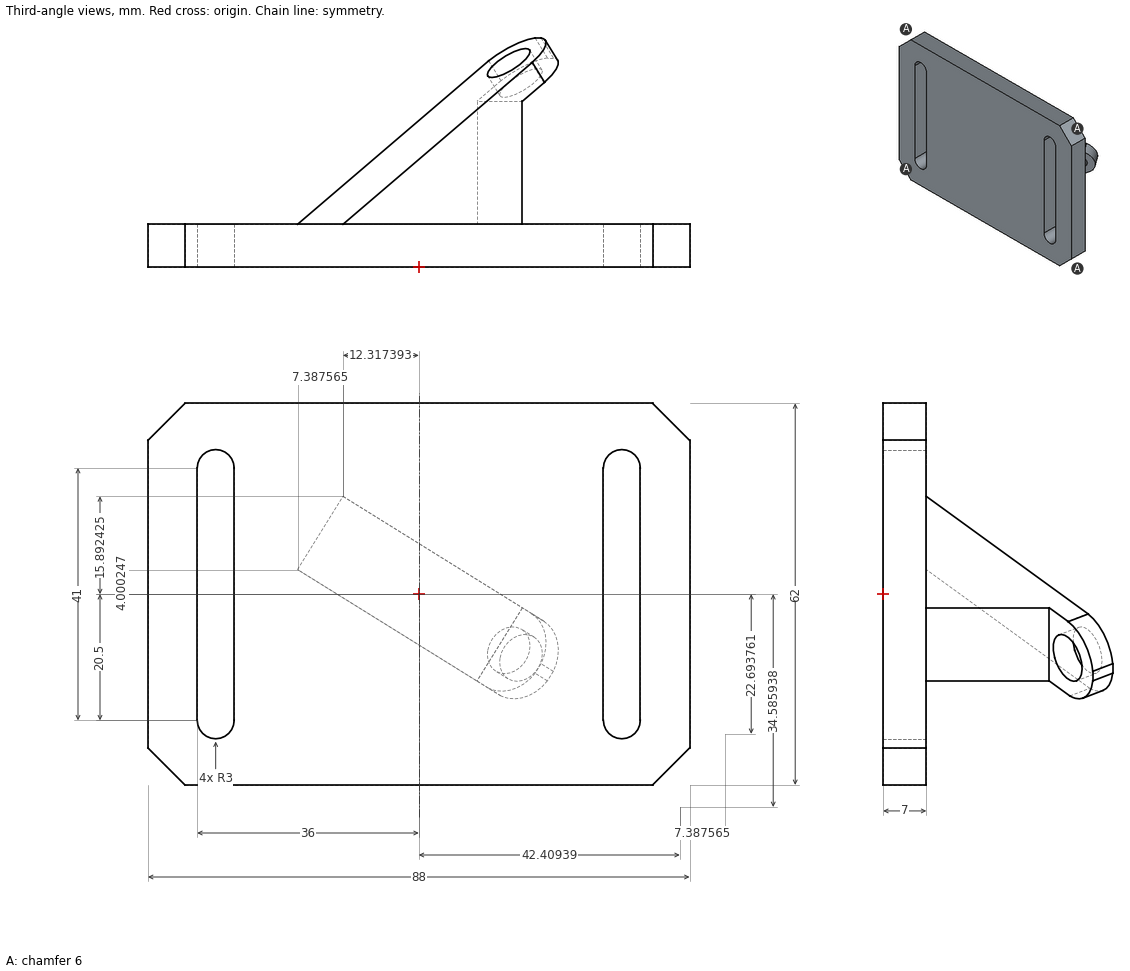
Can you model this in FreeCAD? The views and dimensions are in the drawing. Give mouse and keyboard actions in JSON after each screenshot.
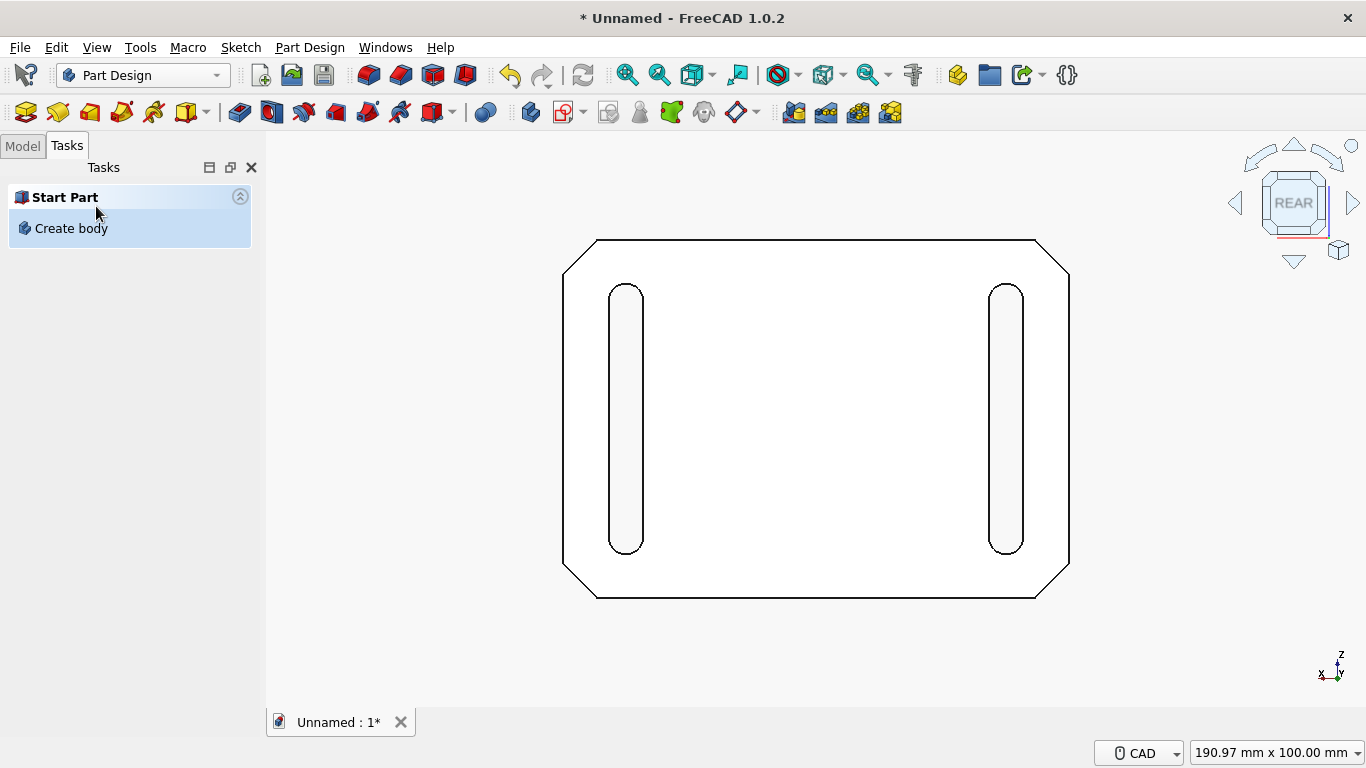
{"action": "left_click", "coordinate": [816, 418]}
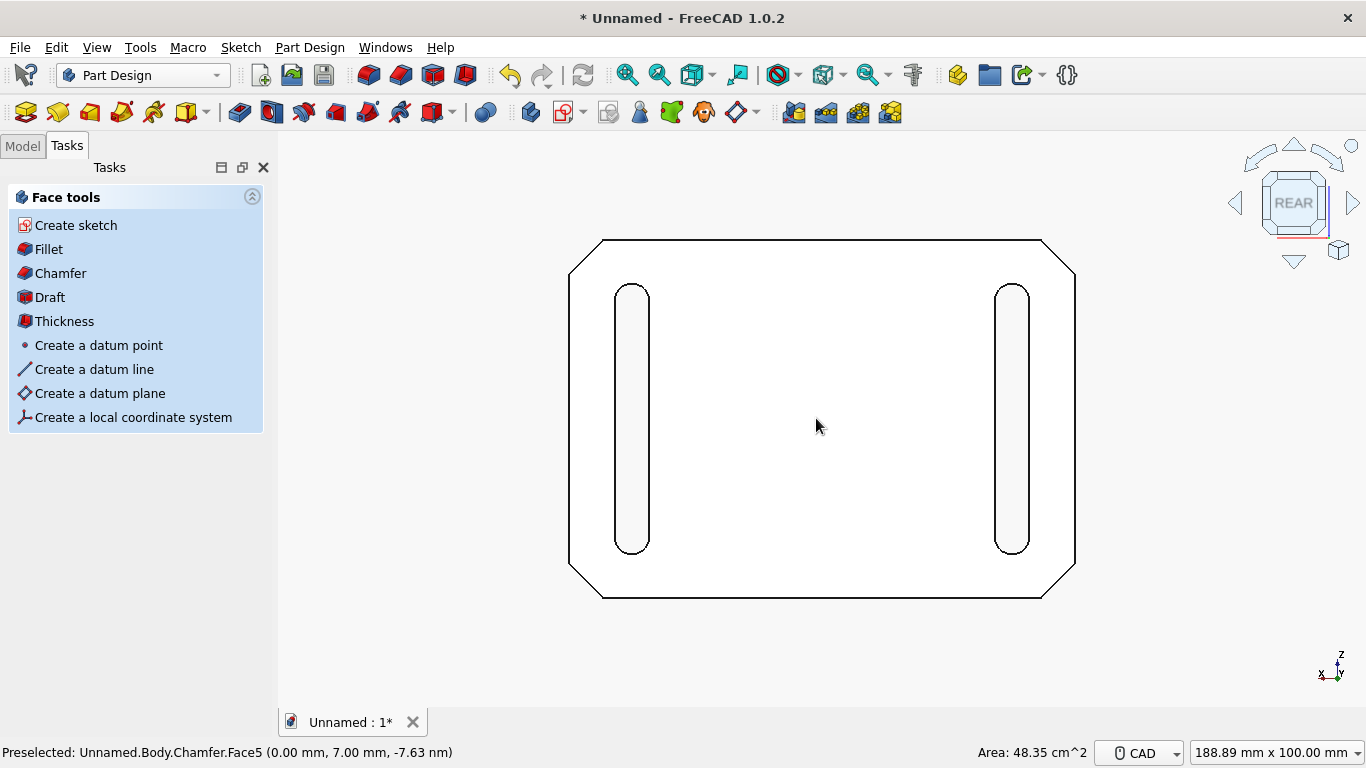
{"action": "left_click", "coordinate": [564, 112]}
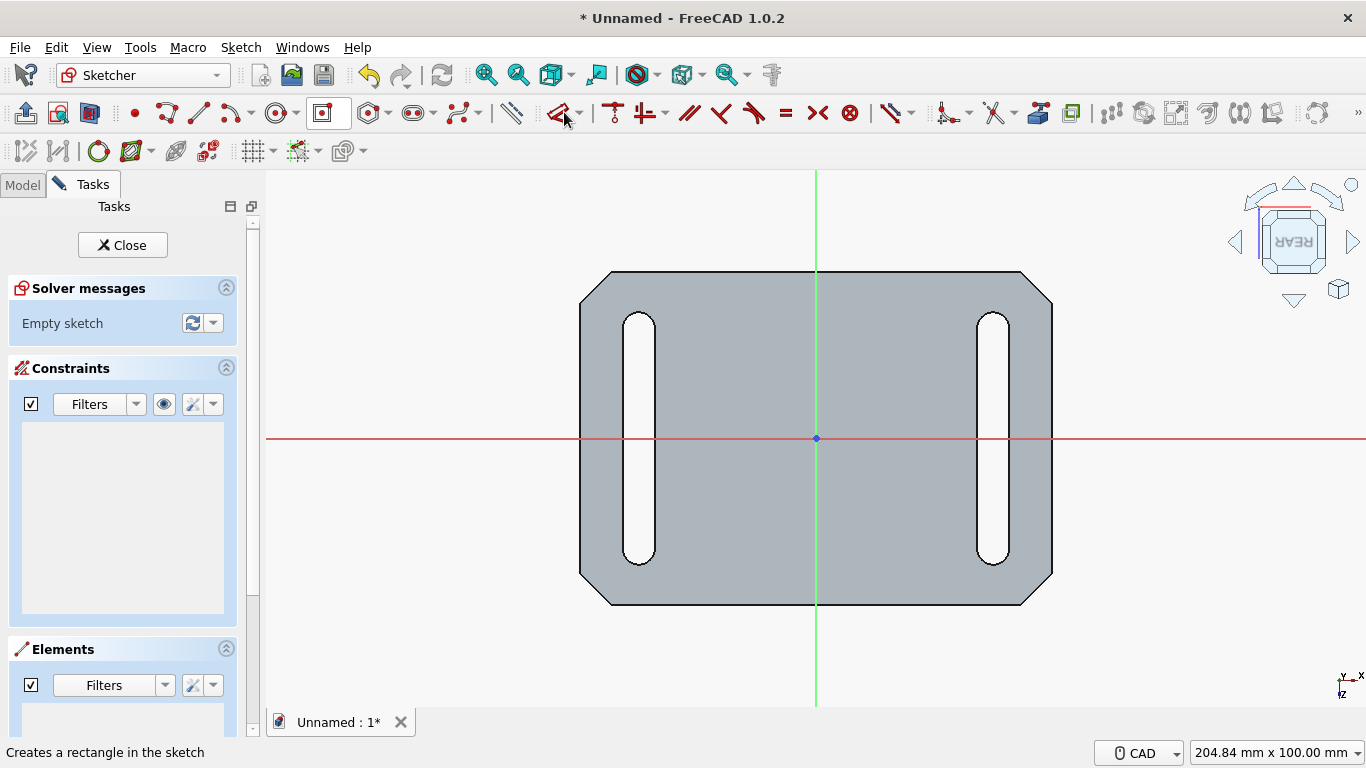
{"action": "left_click", "coordinate": [168, 114]}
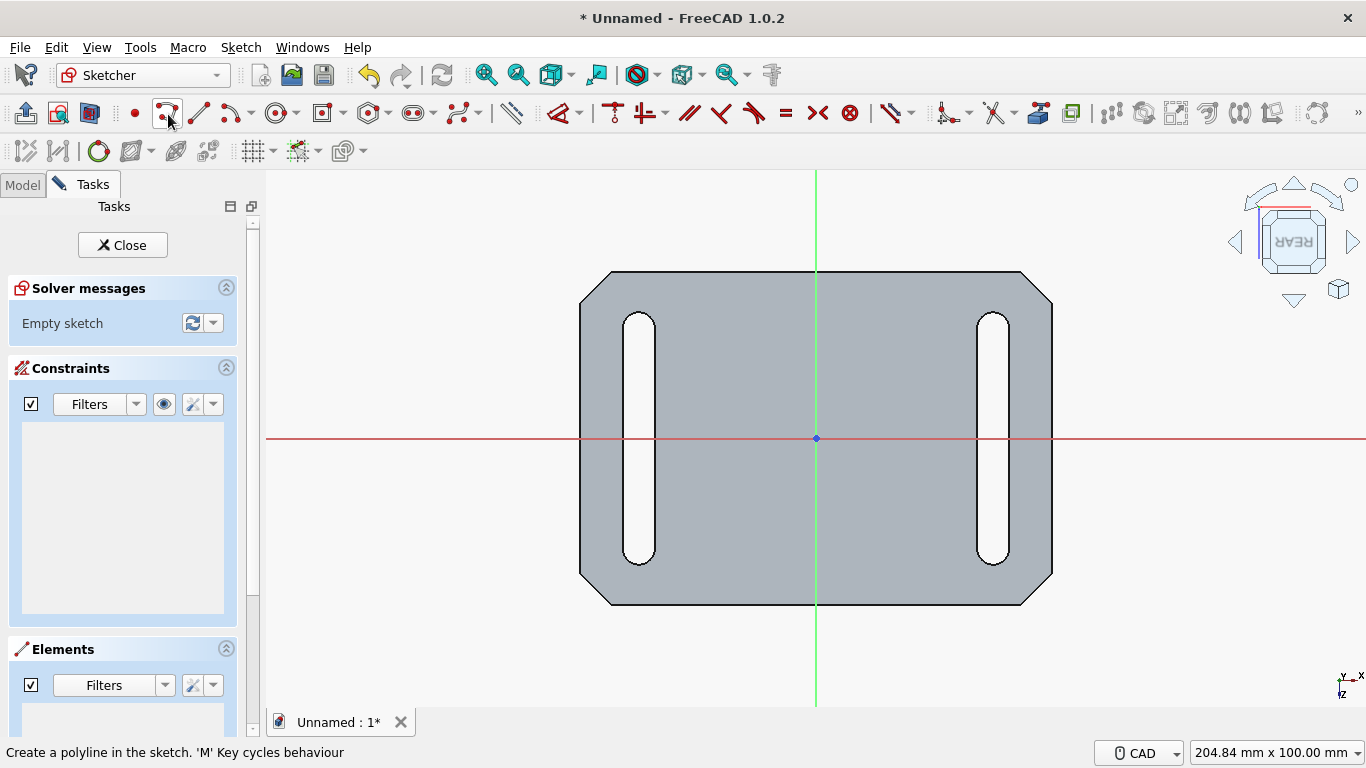
{"action": "left_click", "coordinate": [750, 524]}
{"action": "left_click", "coordinate": [1083, 317]}
{"action": "left_click", "coordinate": [1044, 253]}
{"action": "left_click", "coordinate": [710, 460]}
{"action": "left_click", "coordinate": [750, 525]}
{"action": "key", "text": "Escape"}
{"action": "key", "text": "Escape"}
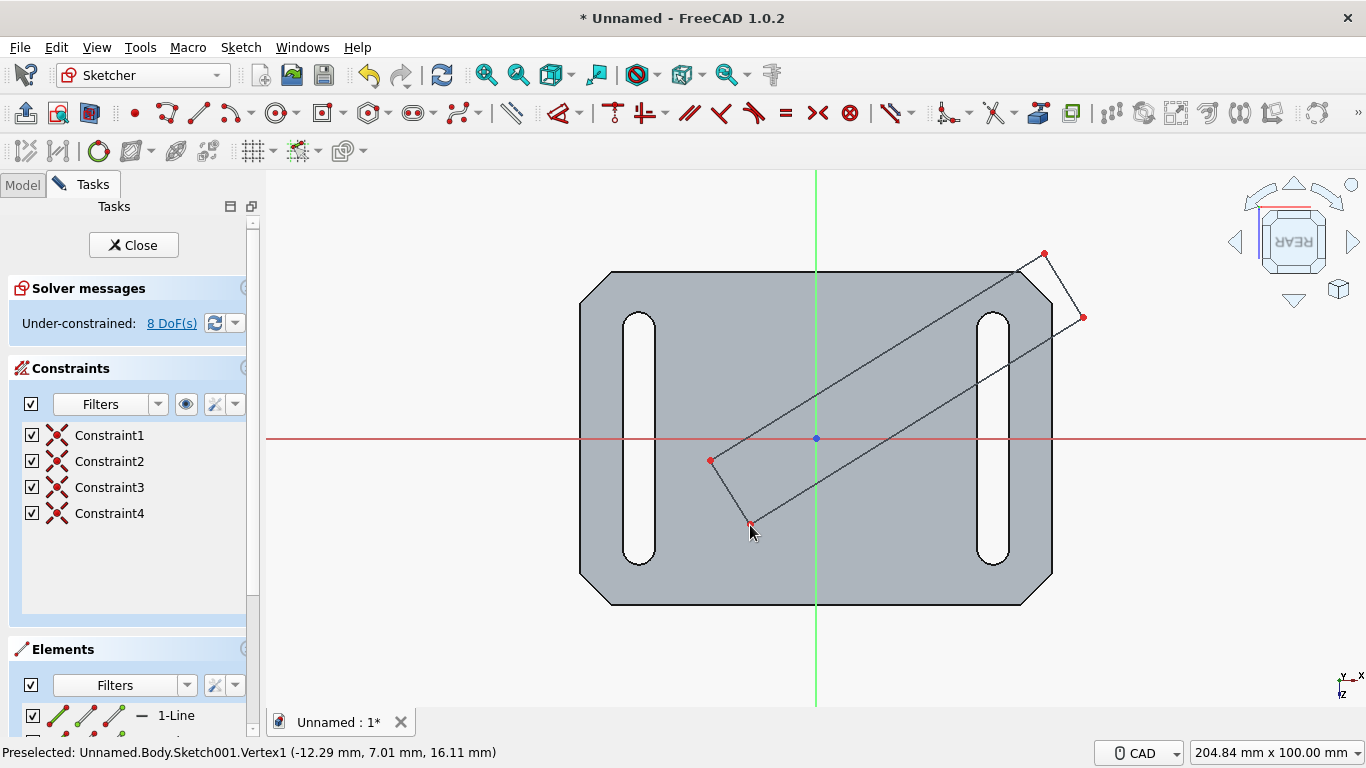
{"action": "left_click", "coordinate": [558, 114]}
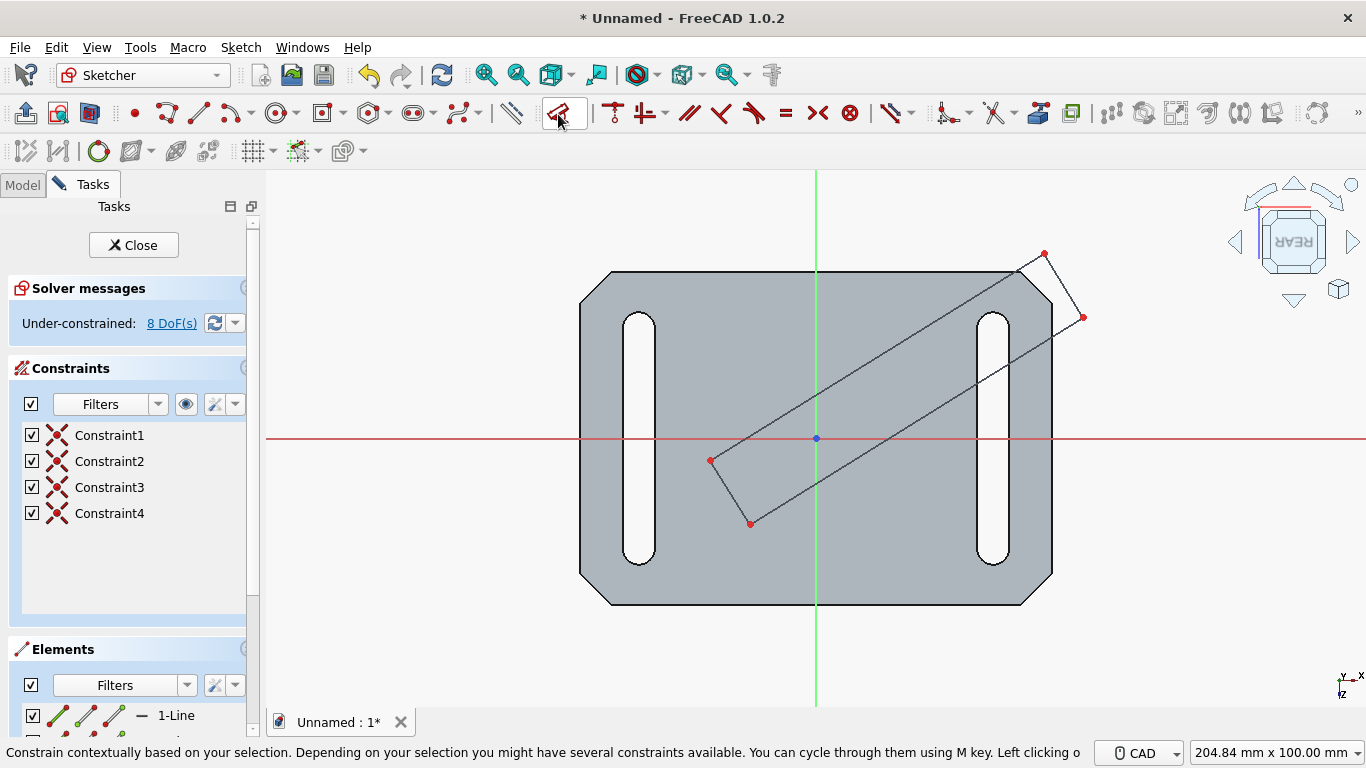
{"action": "left_click", "coordinate": [1044, 254]}
{"action": "left_click", "coordinate": [930, 220]}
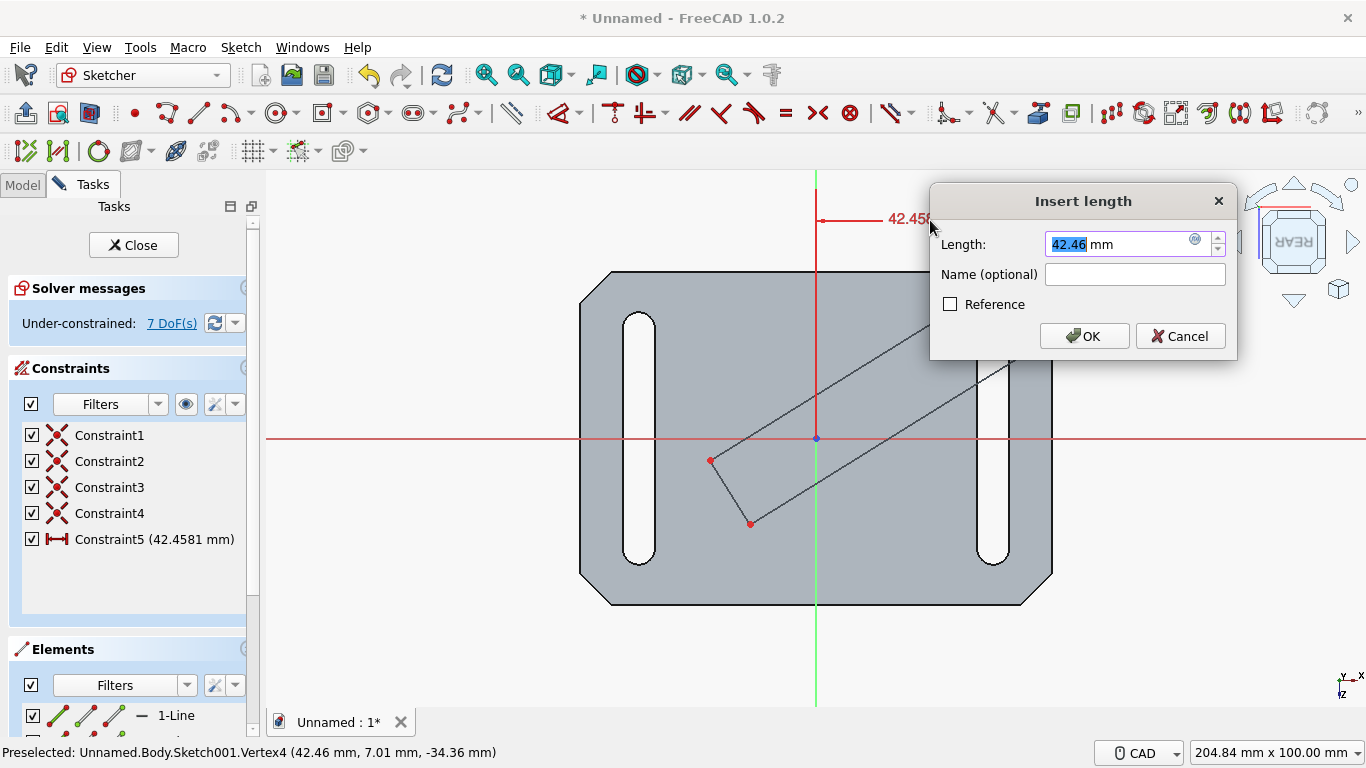
{"action": "type", "text": "42.40939"}
{"action": "key", "text": "Return"}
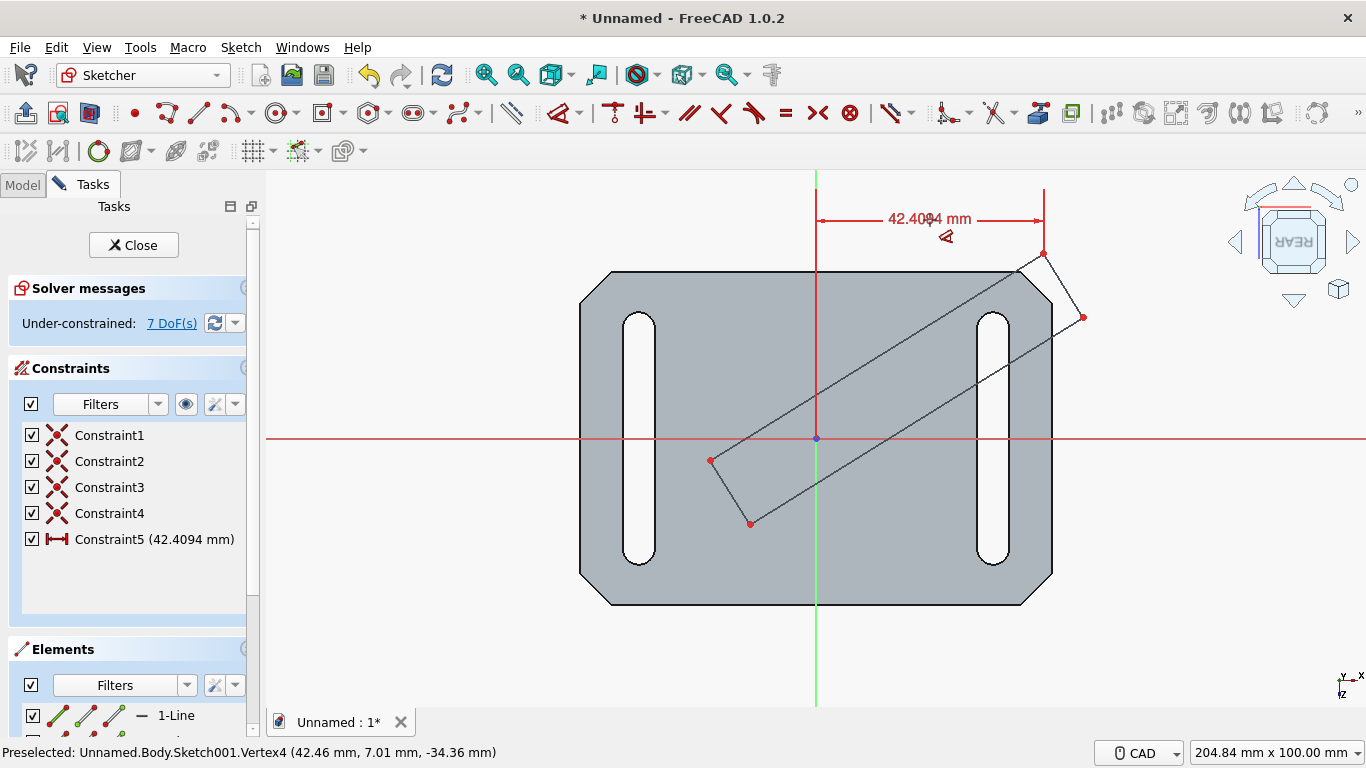
{"action": "scroll", "coordinate": [710, 461], "scroll_direction": "up", "scroll_amount": 4}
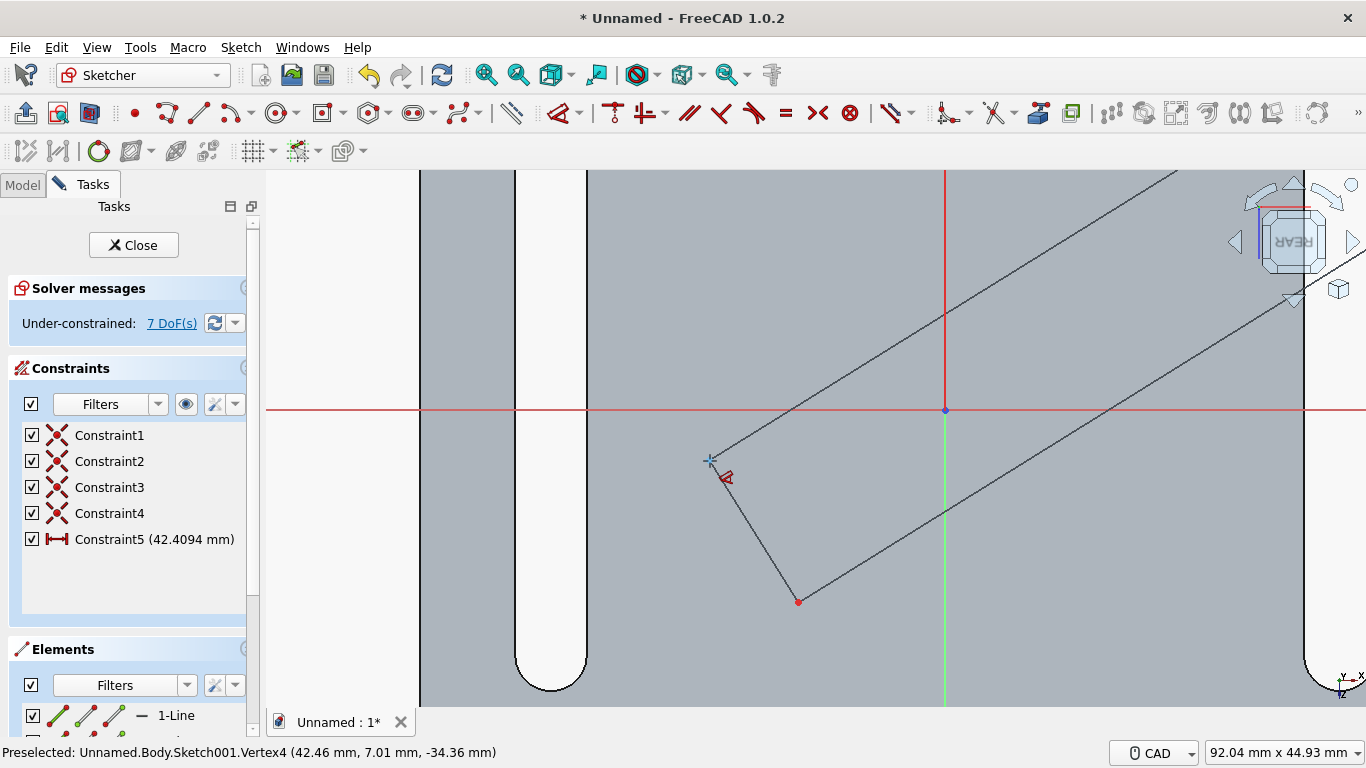
{"action": "left_click", "coordinate": [710, 460]}
{"action": "left_click", "coordinate": [676, 435]}